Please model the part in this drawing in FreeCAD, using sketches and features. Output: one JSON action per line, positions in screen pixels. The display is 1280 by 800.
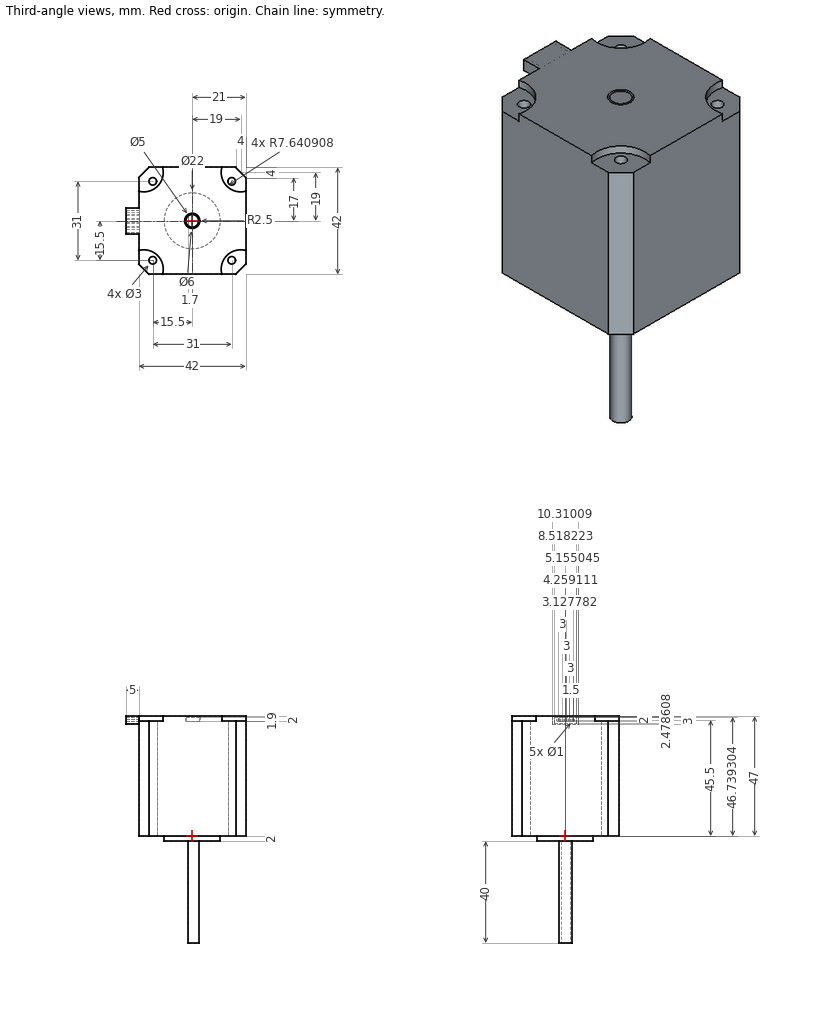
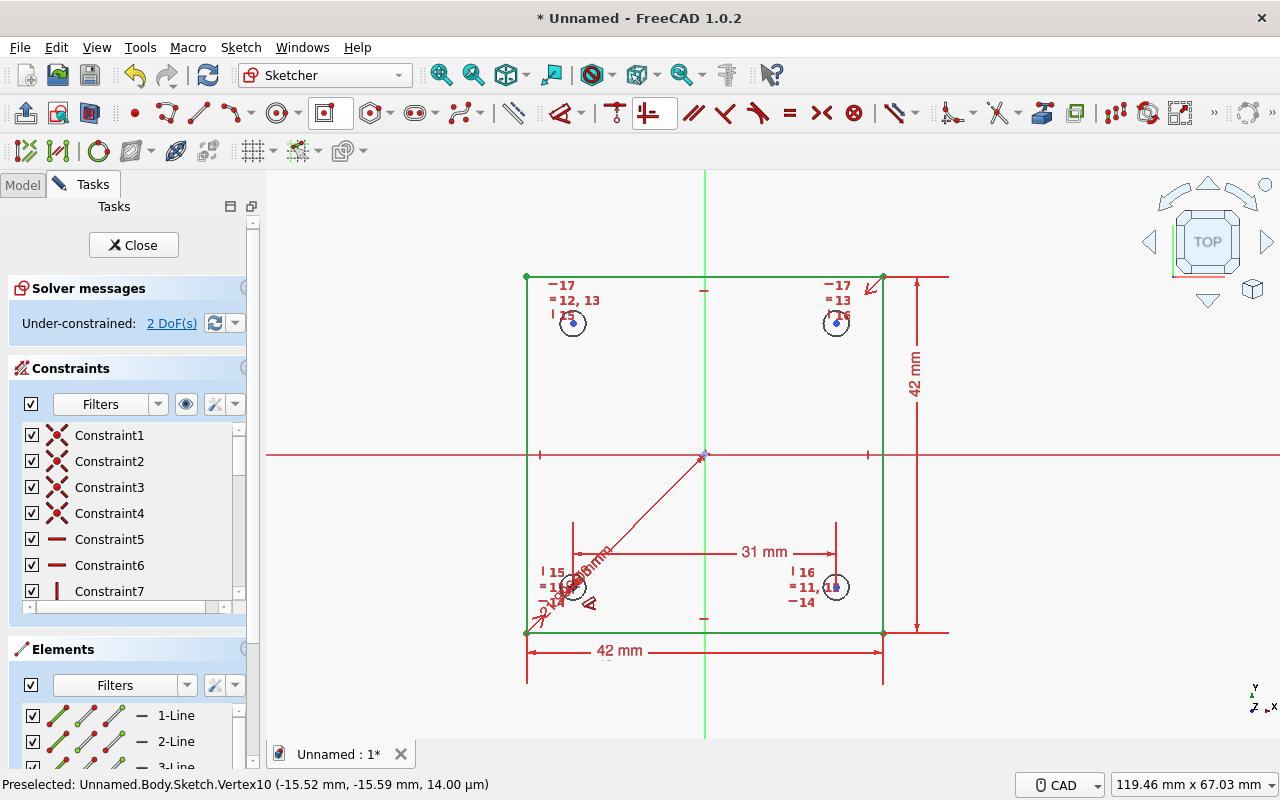
{"action": "left_click", "coordinate": [573, 324]}
{"action": "left_click", "coordinate": [607, 395]}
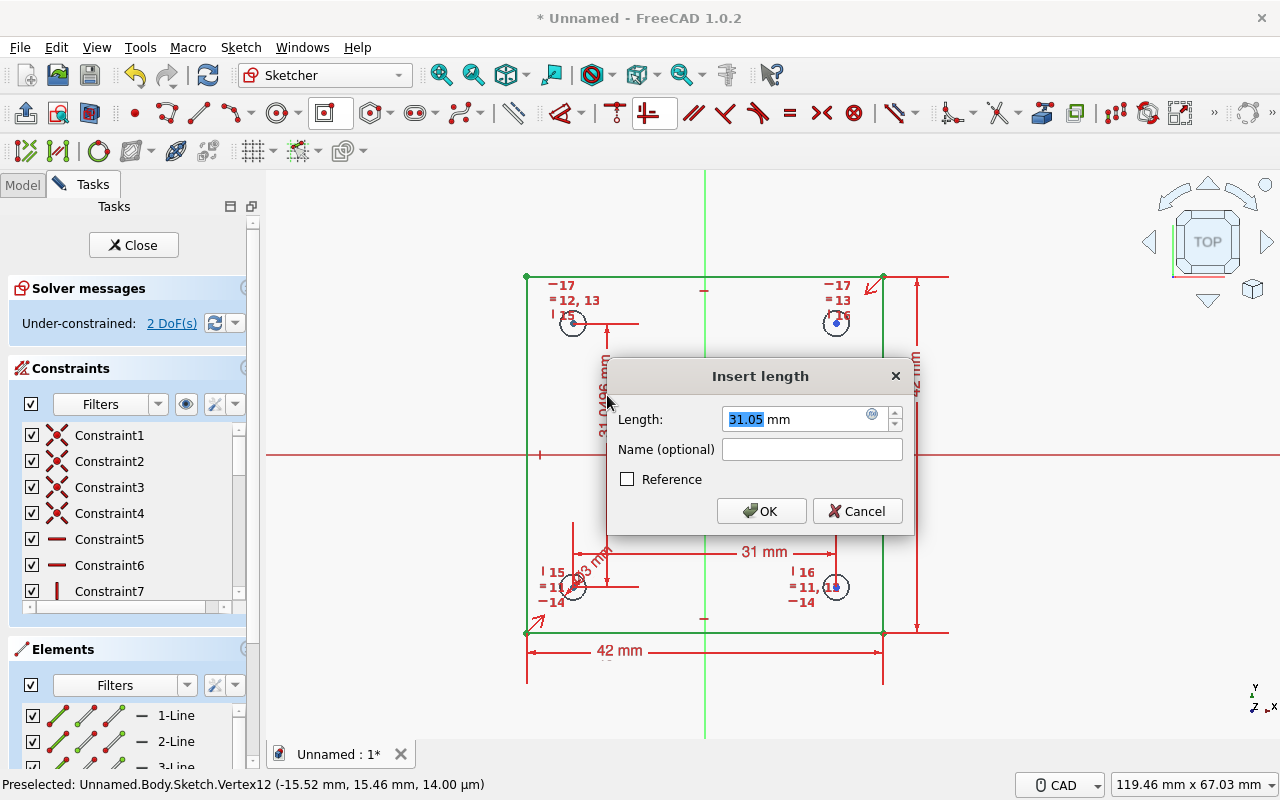
{"action": "type", "text": "31"}
{"action": "key", "text": "Return"}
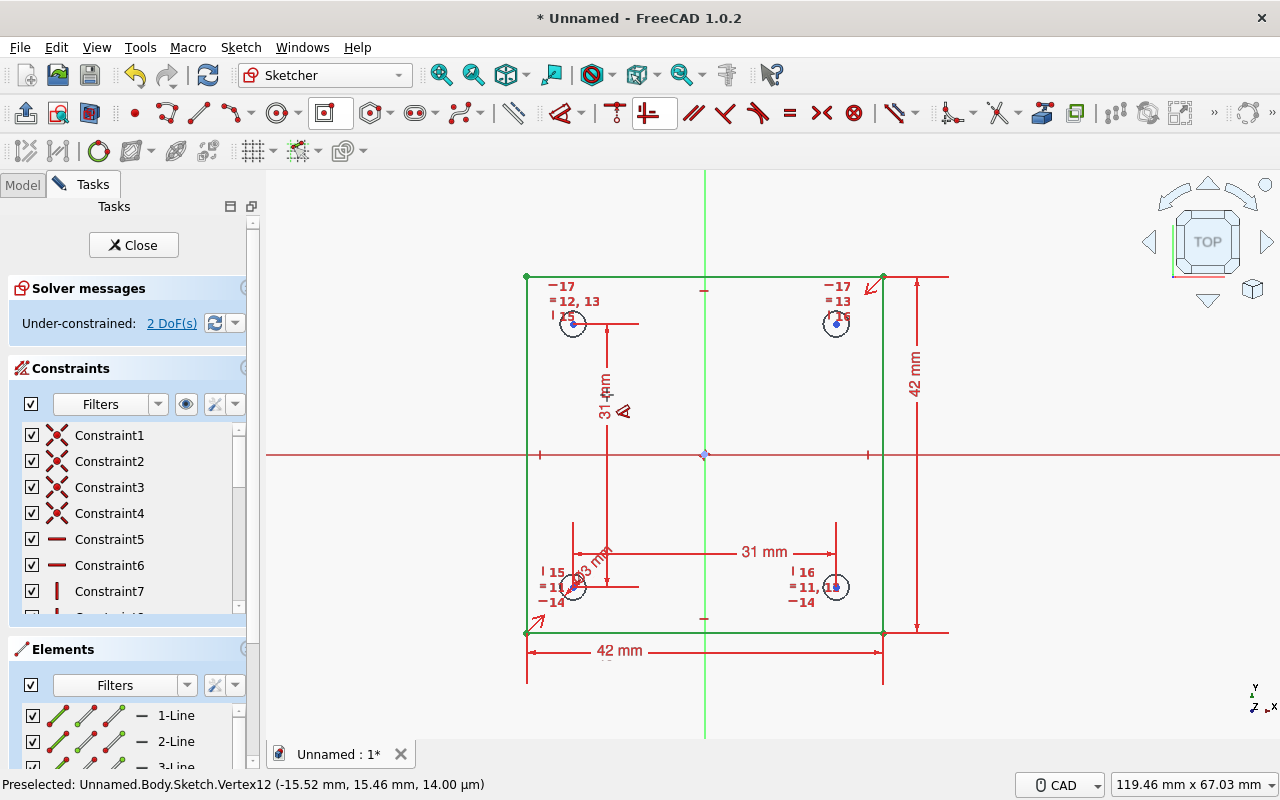
{"action": "left_click", "coordinate": [573, 587]}
{"action": "left_click", "coordinate": [639, 421]}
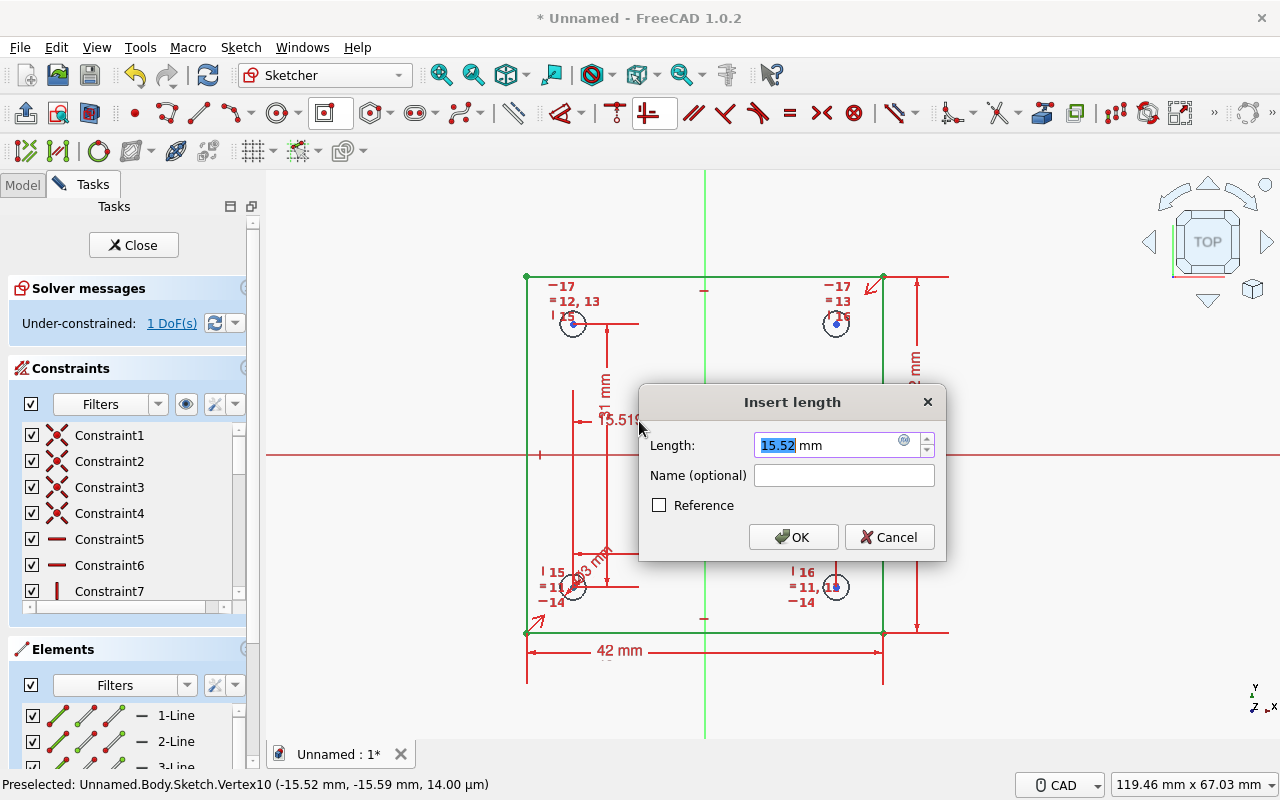
{"action": "type", "text": "15.5"}
{"action": "key", "text": "Return"}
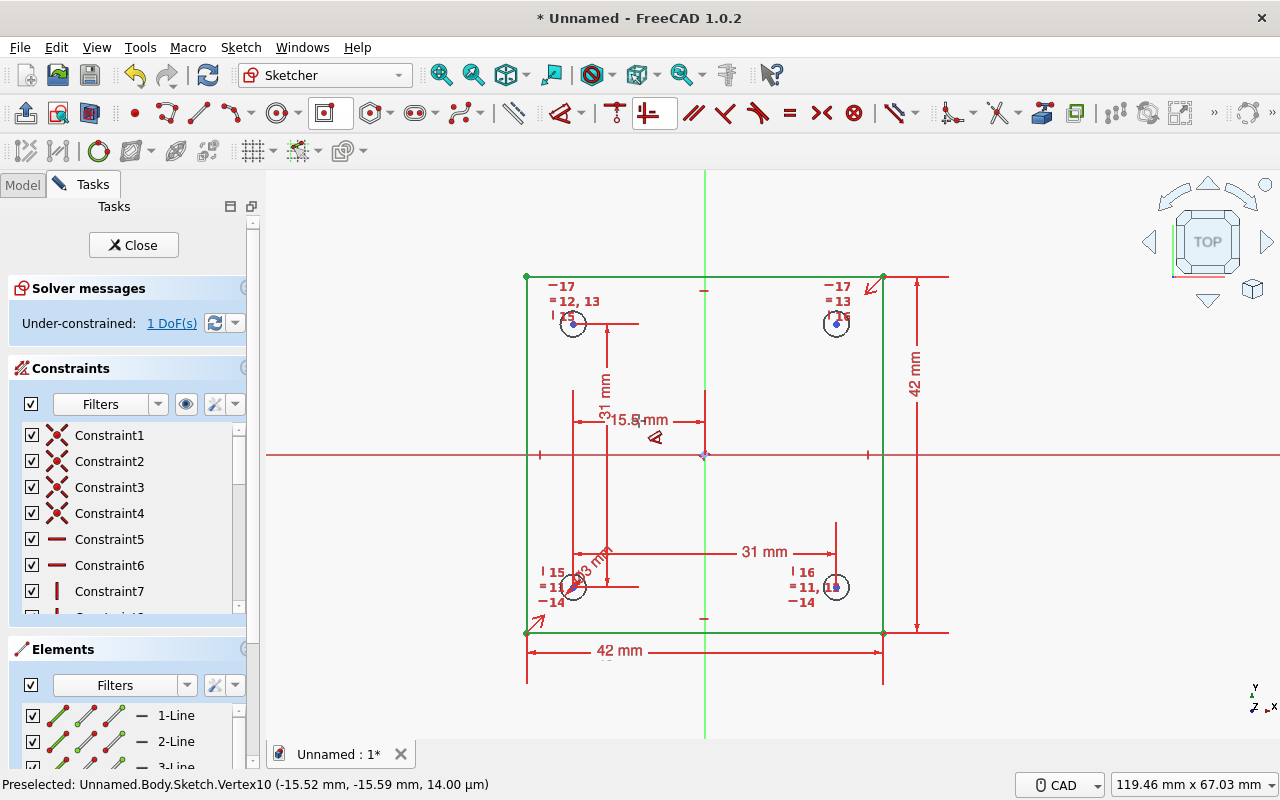
{"action": "left_click", "coordinate": [573, 587]}
{"action": "left_click", "coordinate": [739, 521]}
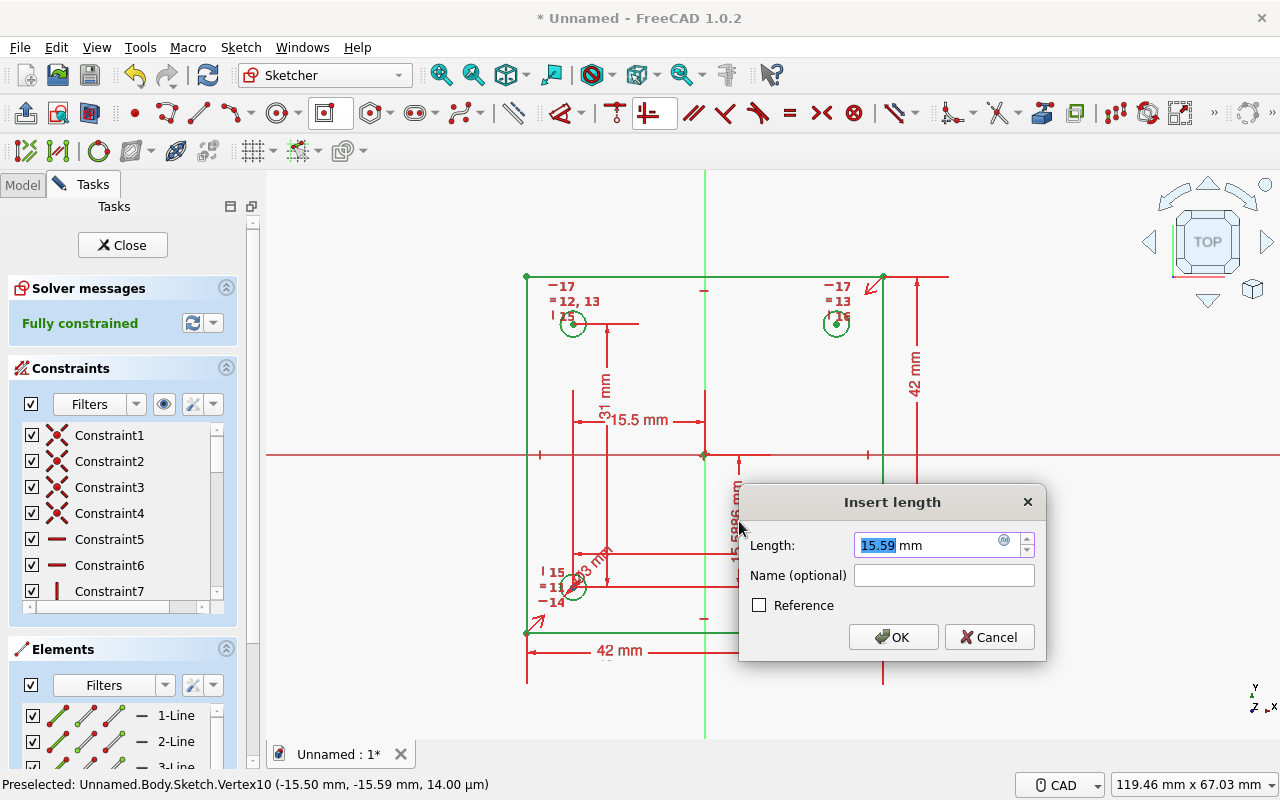
{"action": "type", "text": "15.5"}
{"action": "key", "text": "Return"}
{"action": "key", "text": "Escape"}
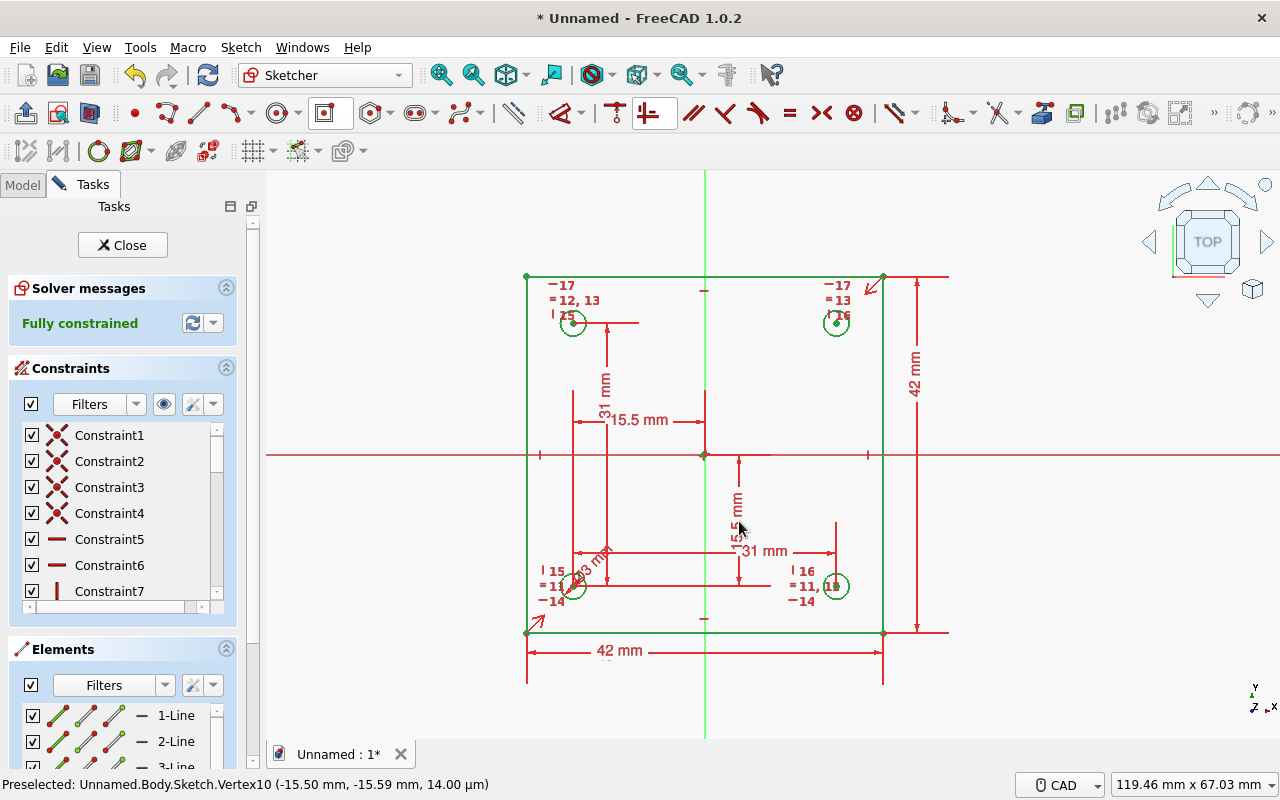
{"action": "left_click", "coordinate": [123, 245]}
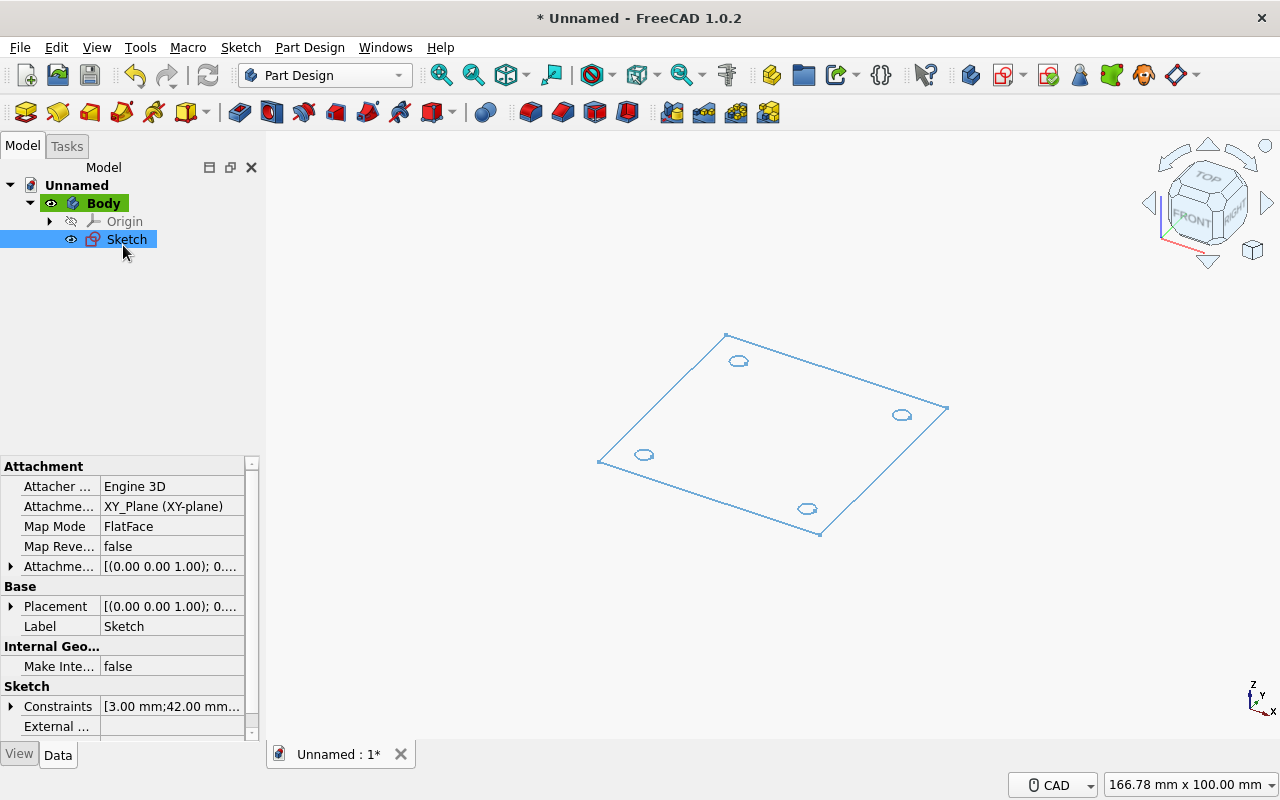
{"action": "left_click", "coordinate": [26, 112]}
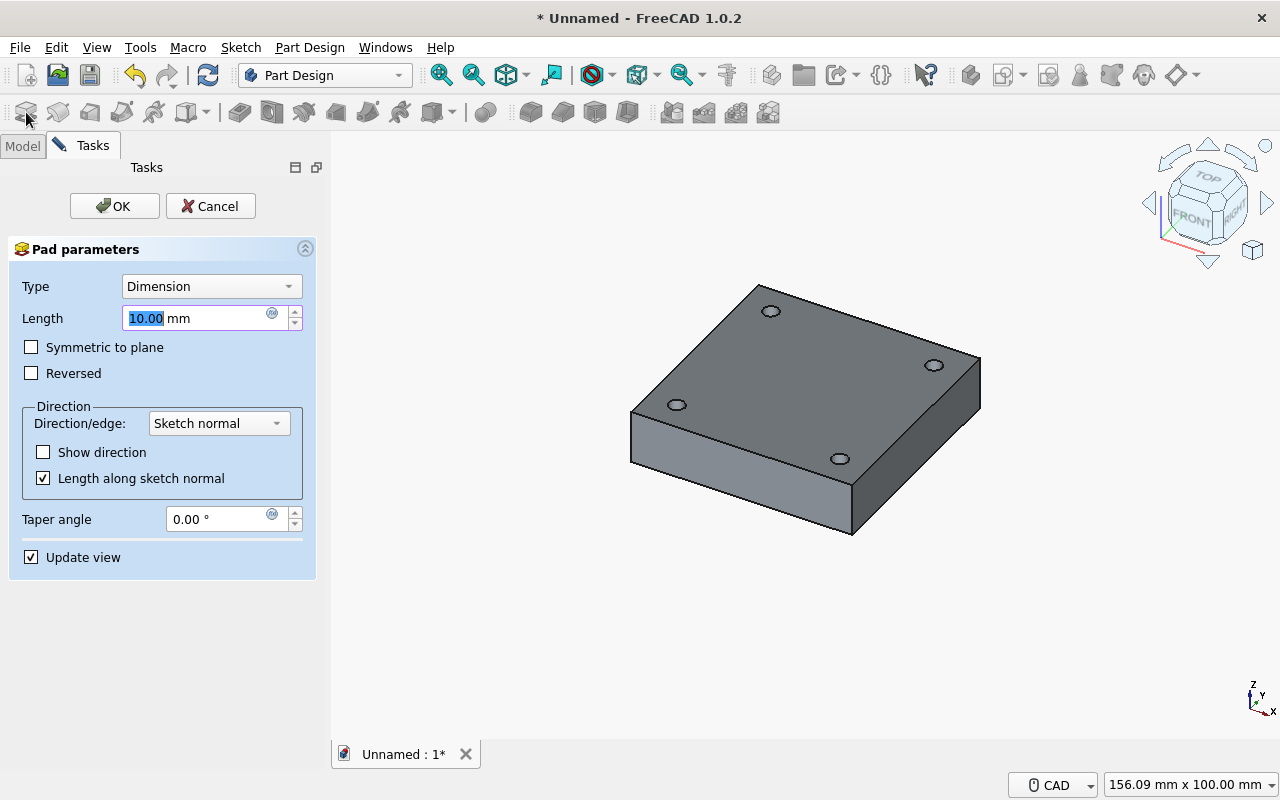
{"action": "type", "text": "47"}
{"action": "key", "text": "Tab"}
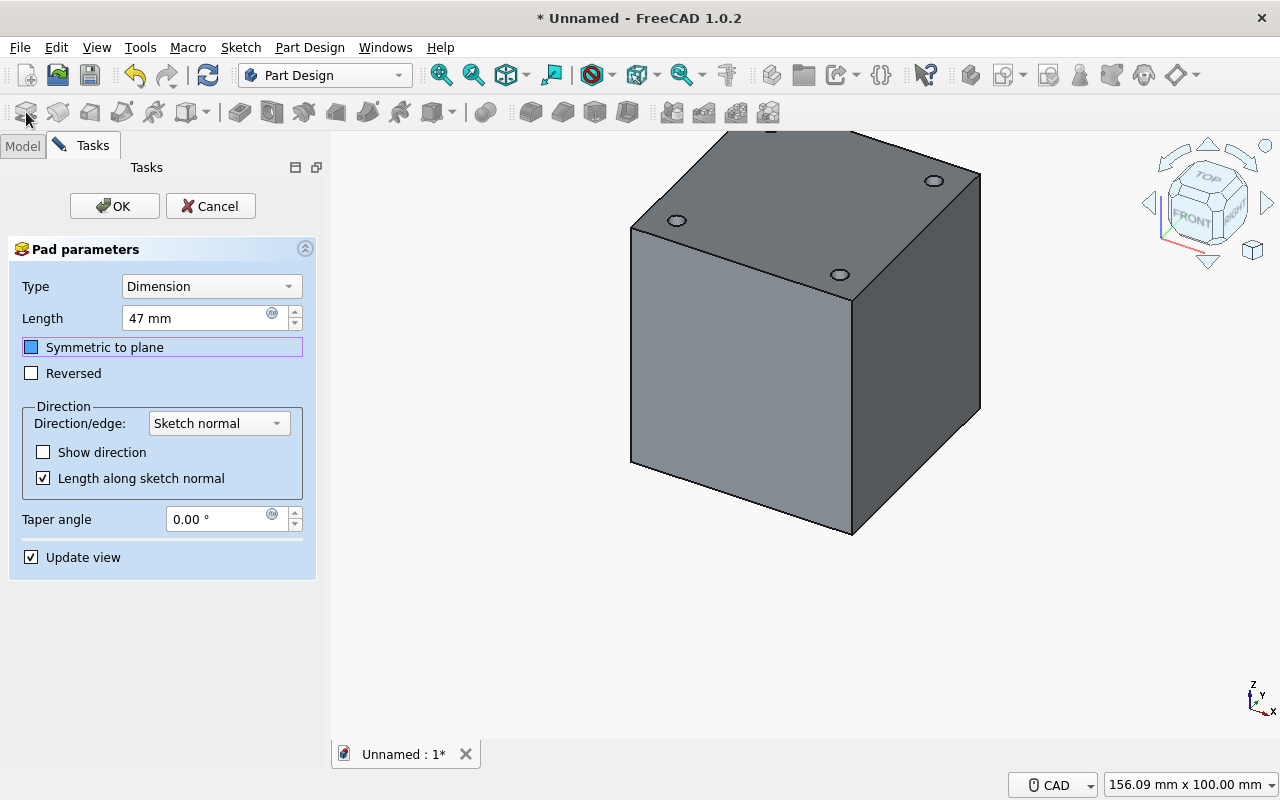
{"action": "left_click", "coordinate": [115, 206]}